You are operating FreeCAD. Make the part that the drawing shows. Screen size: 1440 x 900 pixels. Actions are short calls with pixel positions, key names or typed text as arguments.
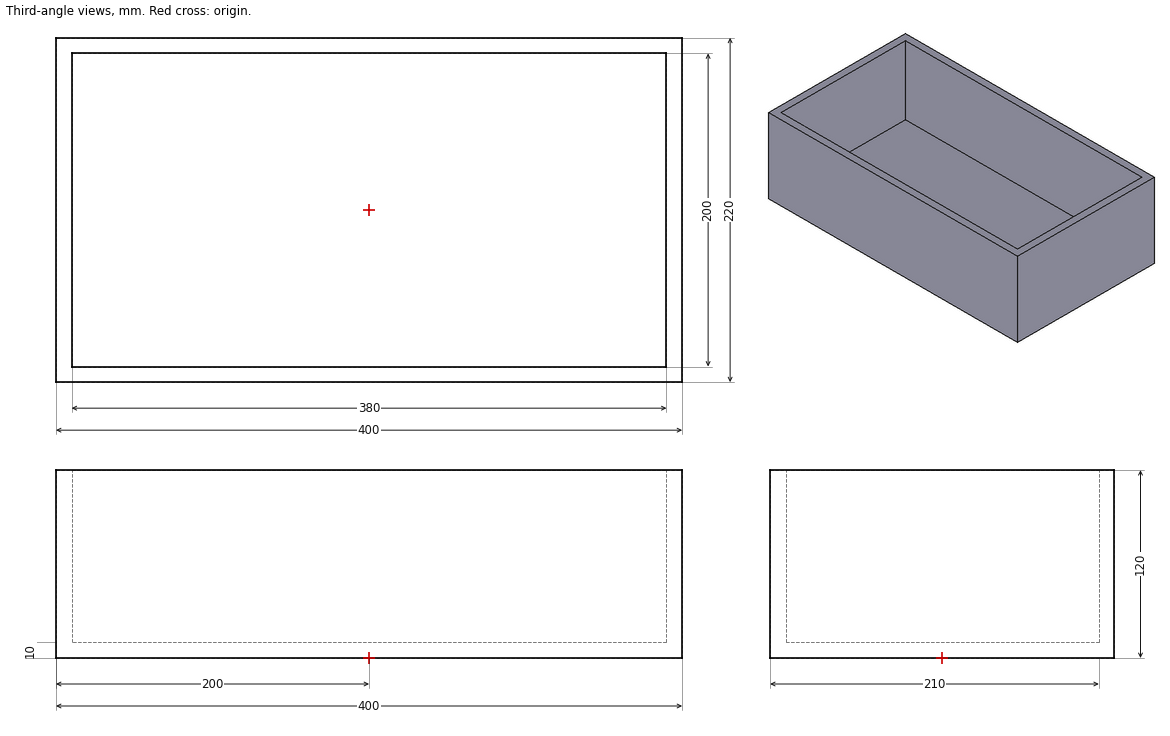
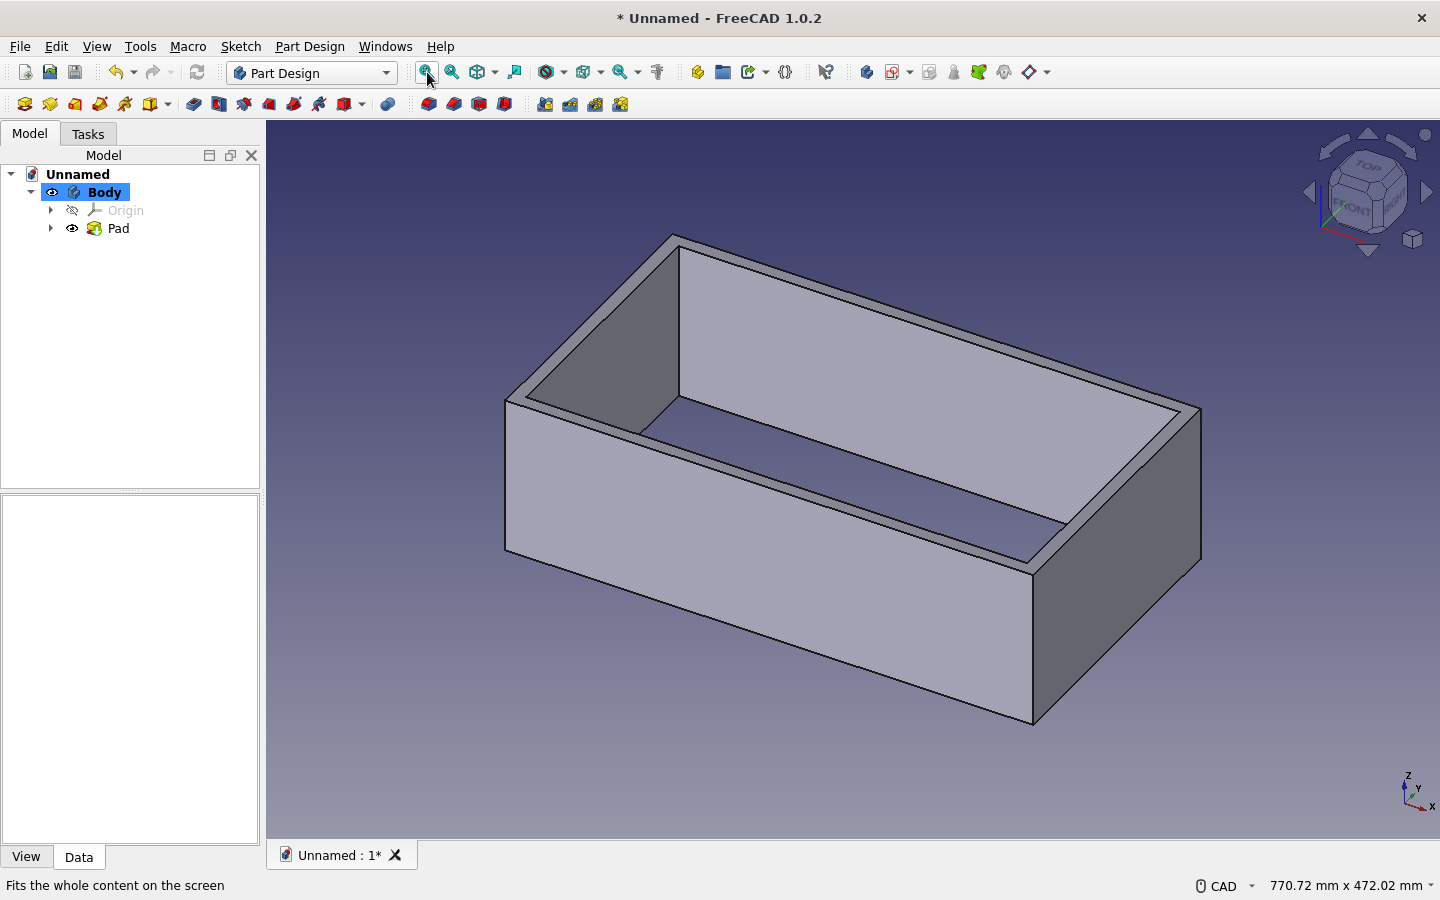
click(51, 210)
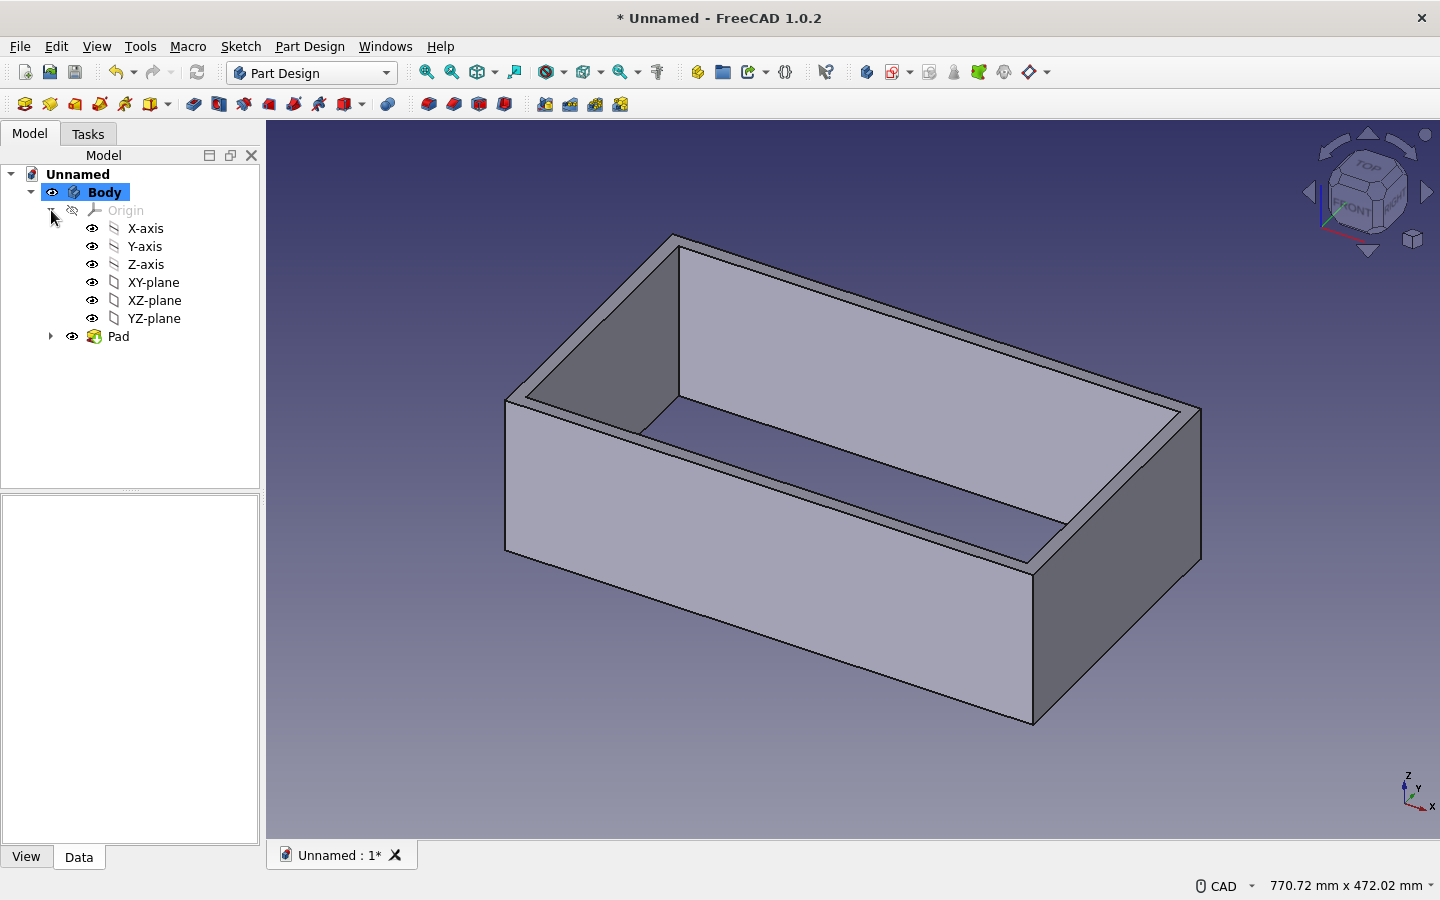
click(137, 300)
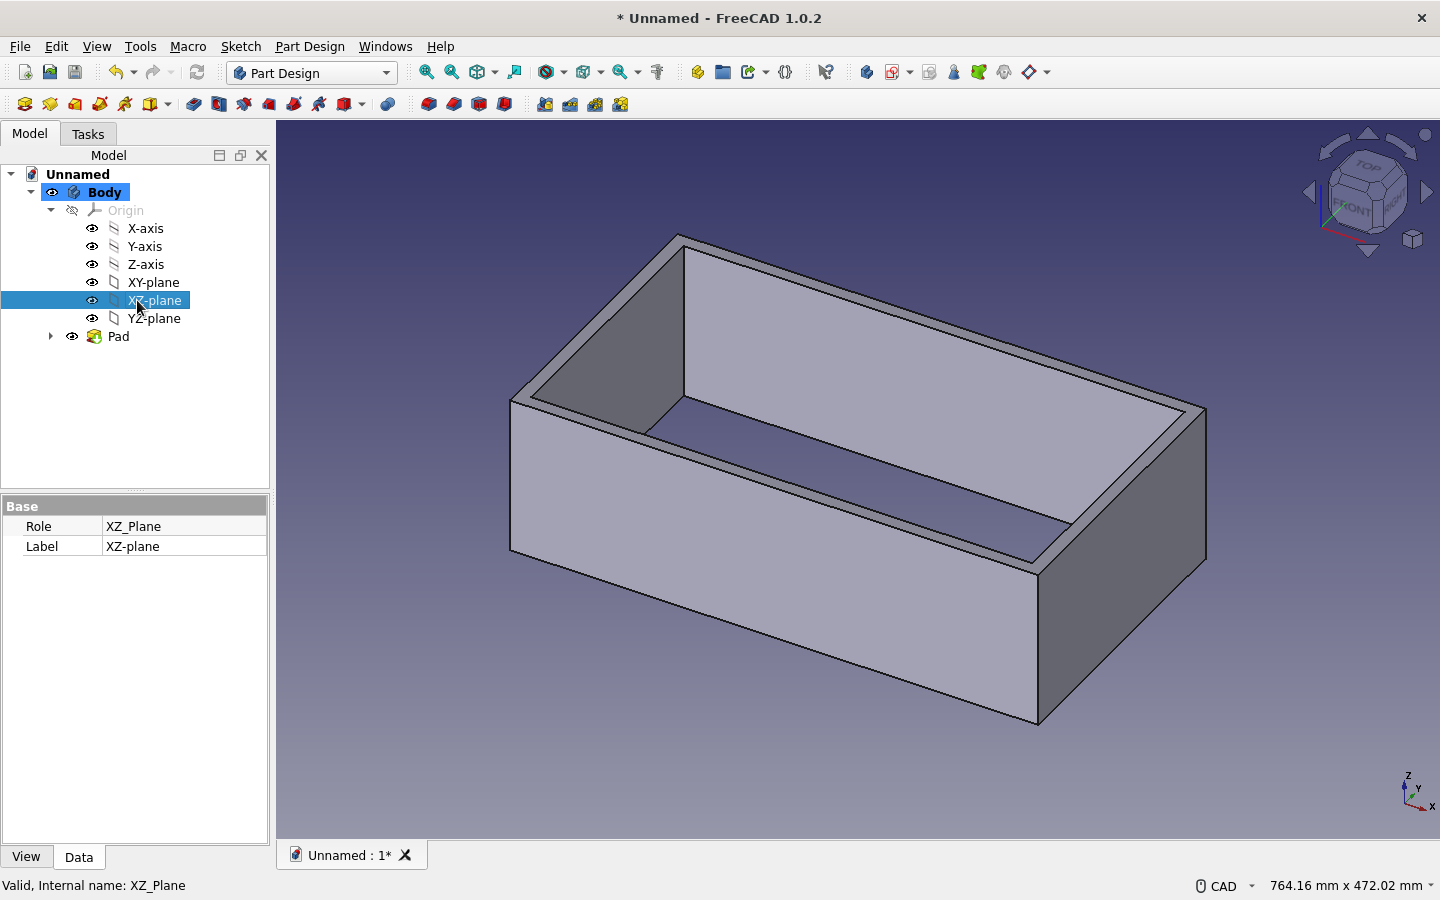
click(1028, 72)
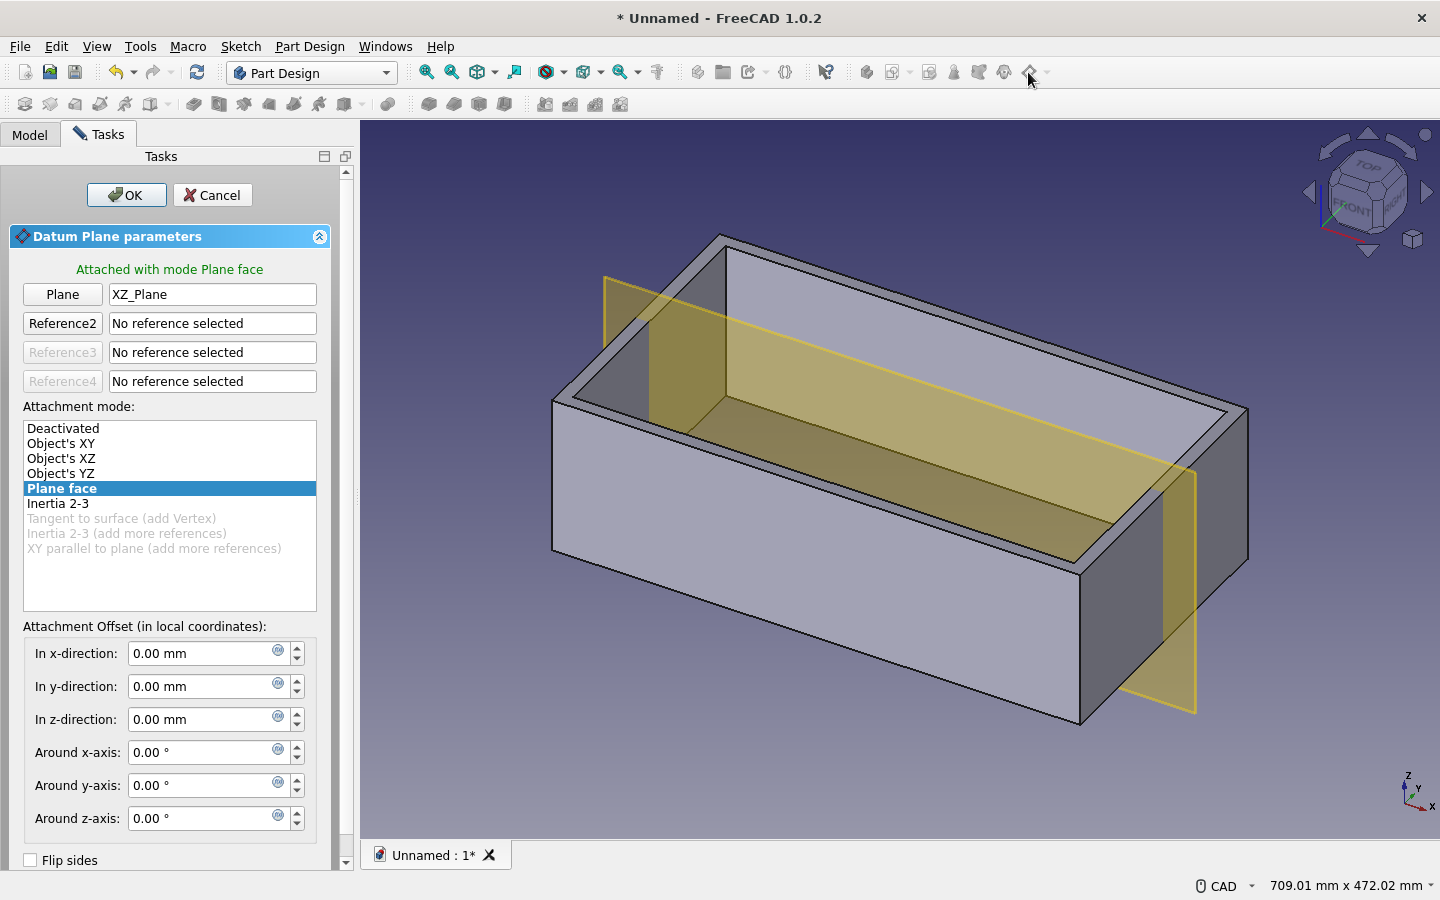
triple_click(210, 720)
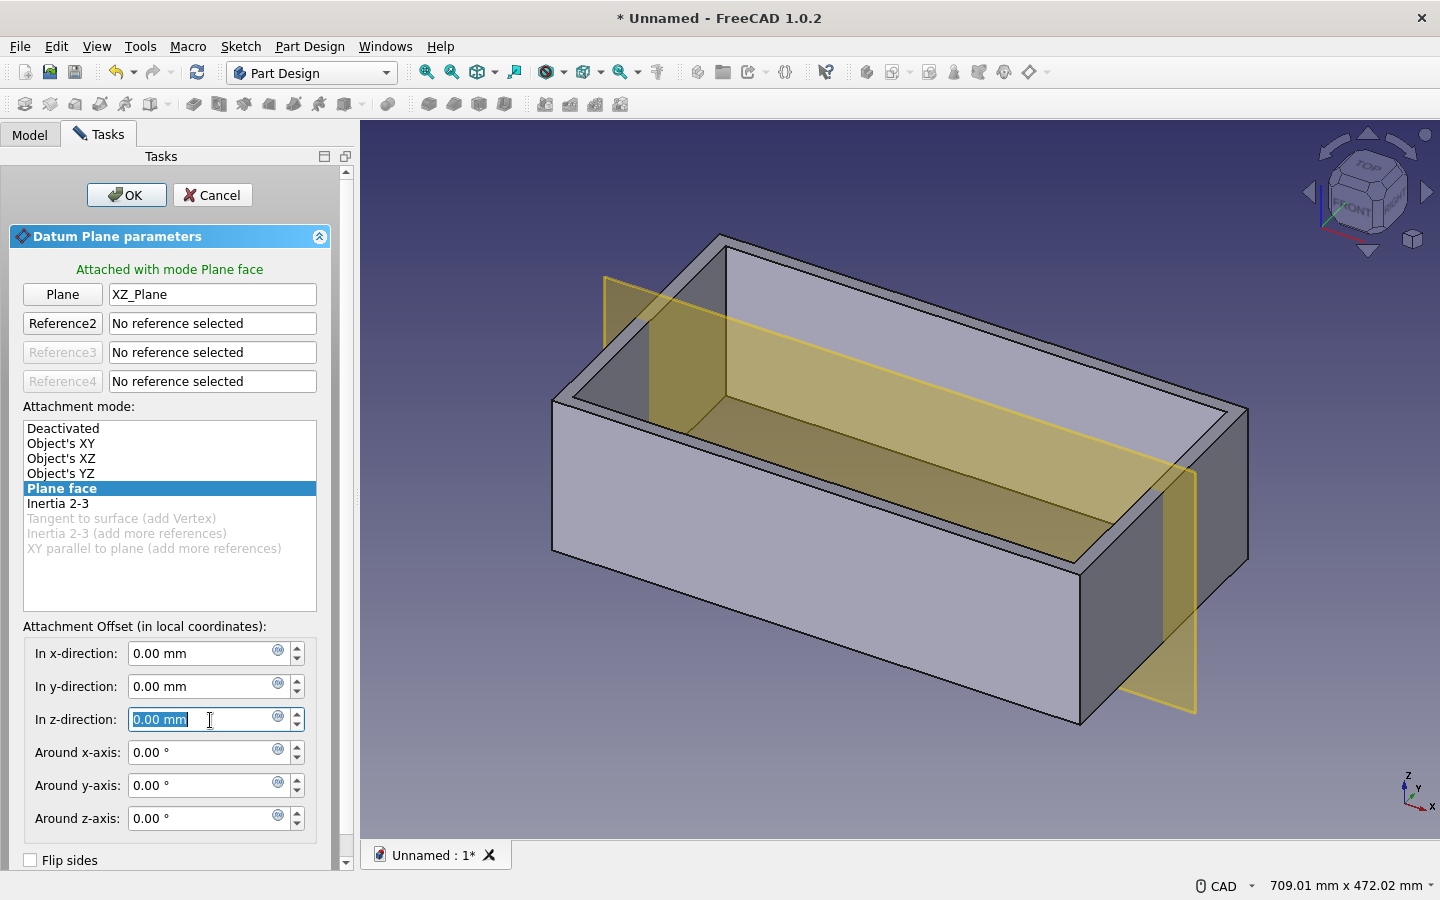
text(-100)
key(Tab)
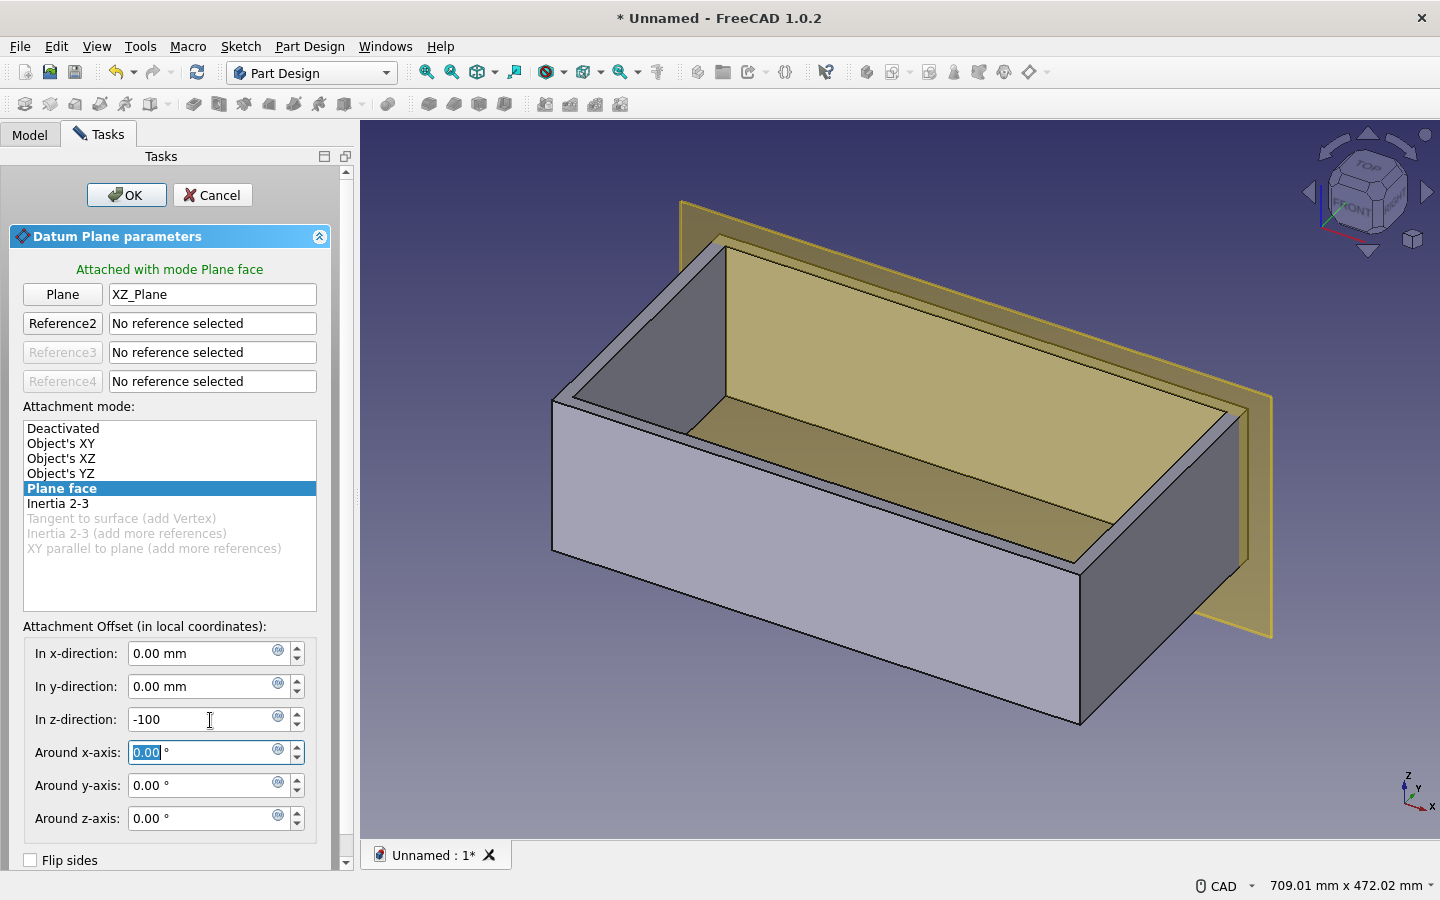
click(127, 195)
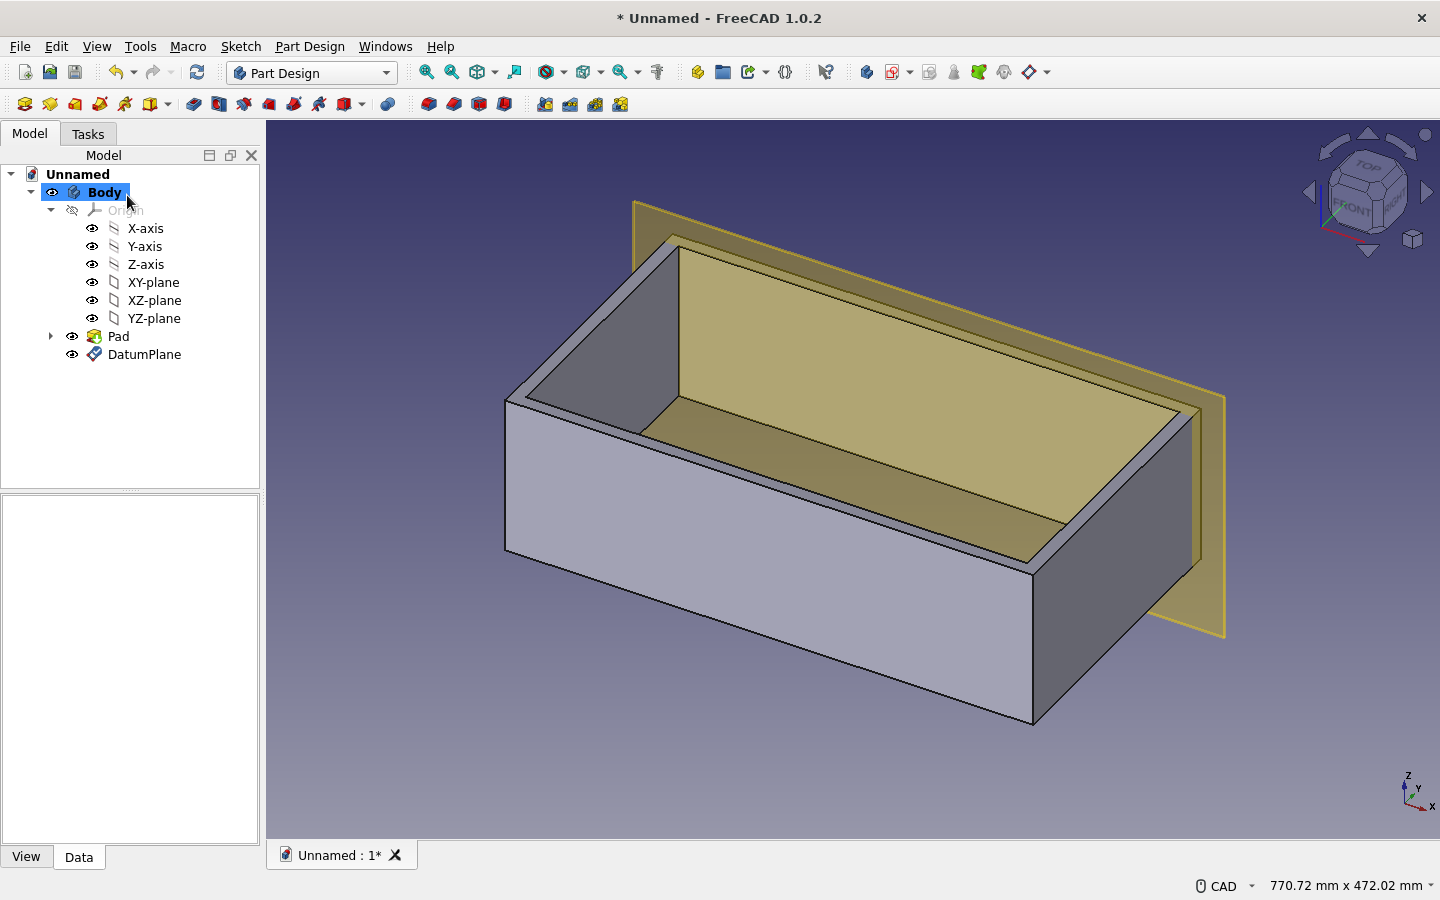
click(117, 354)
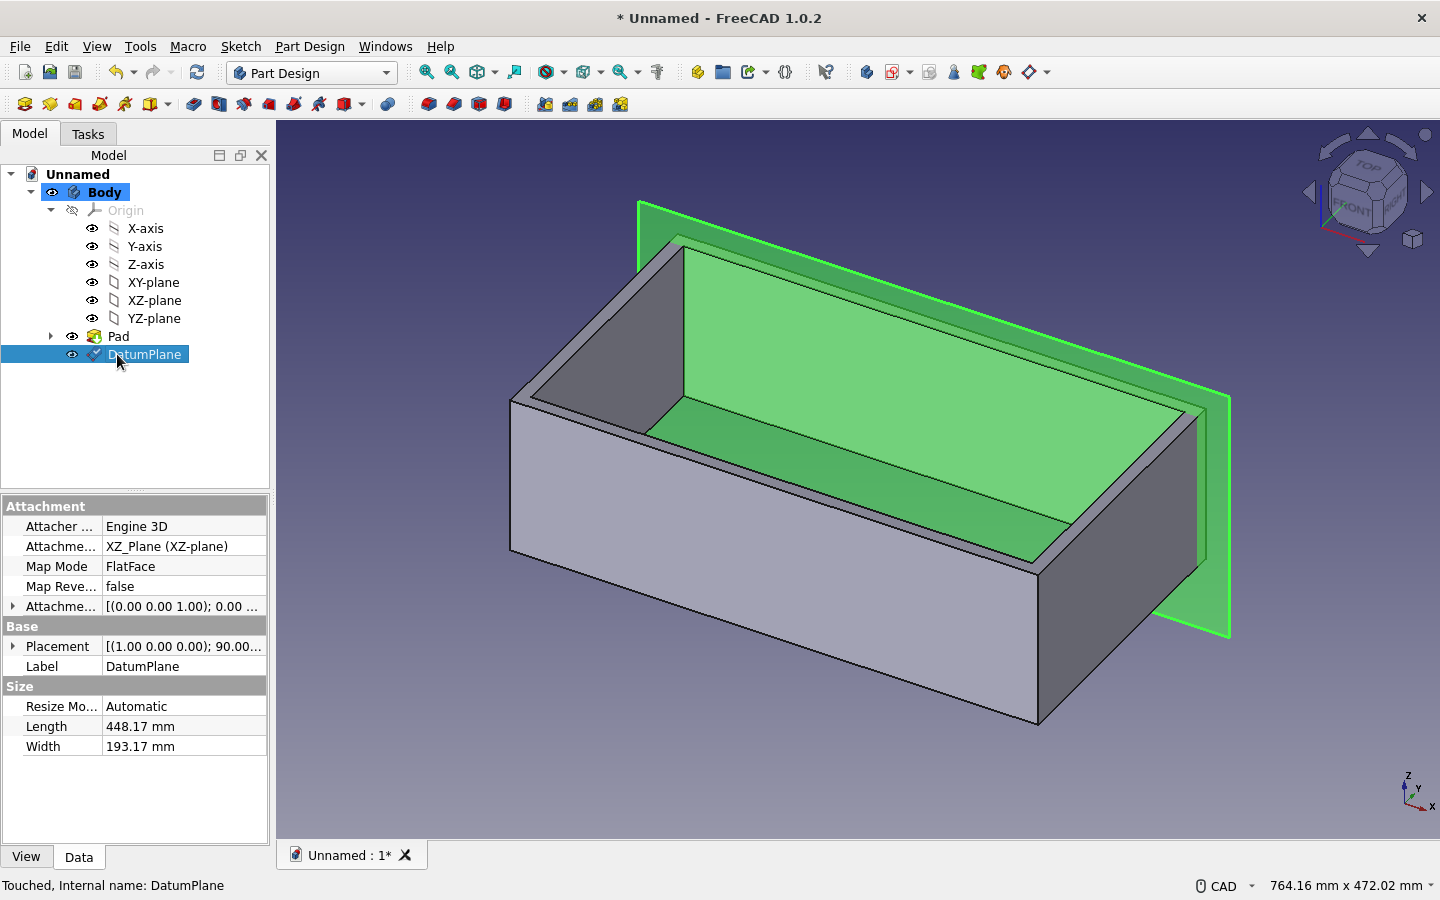
click(892, 72)